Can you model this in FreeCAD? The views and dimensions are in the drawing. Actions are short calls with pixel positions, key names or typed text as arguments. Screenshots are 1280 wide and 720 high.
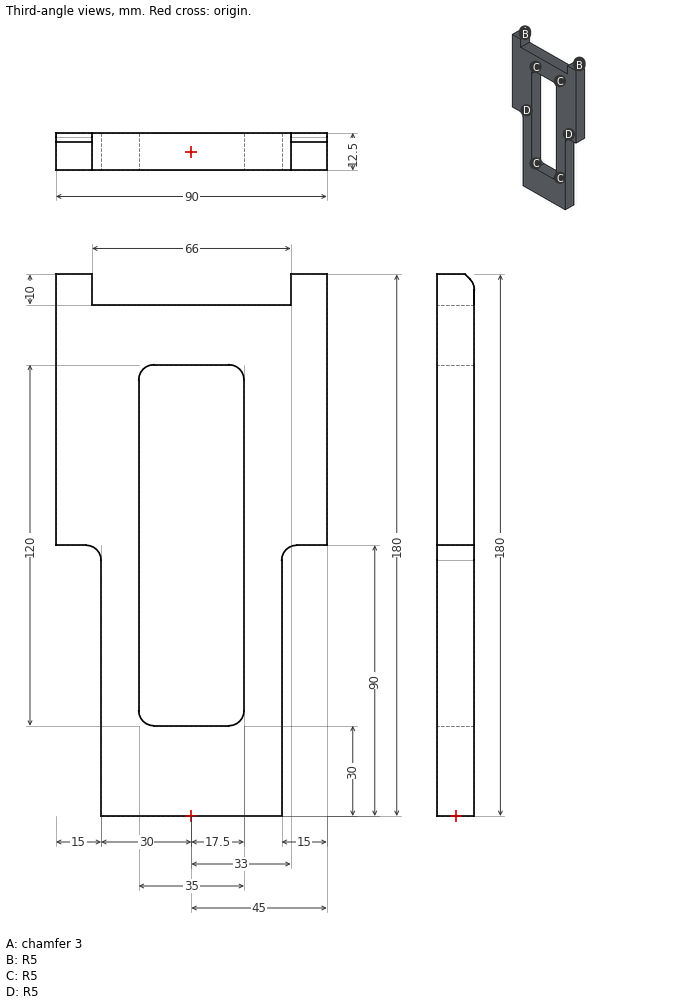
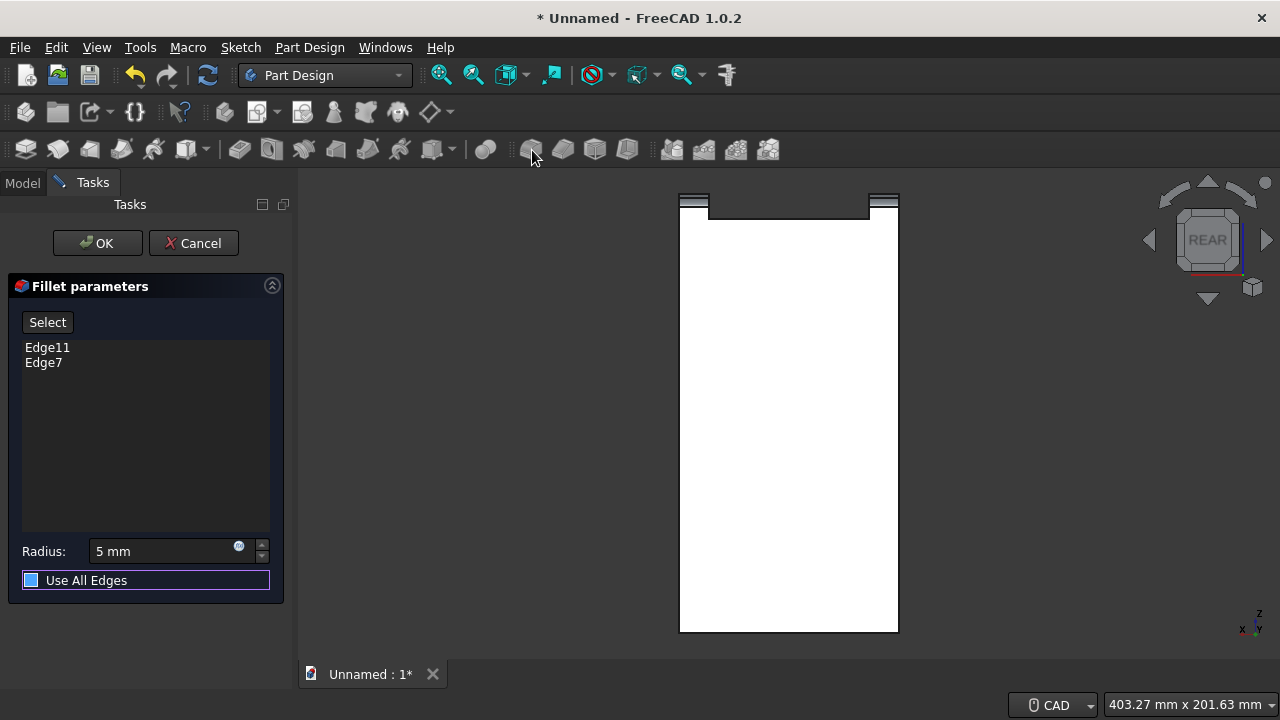
click(98, 243)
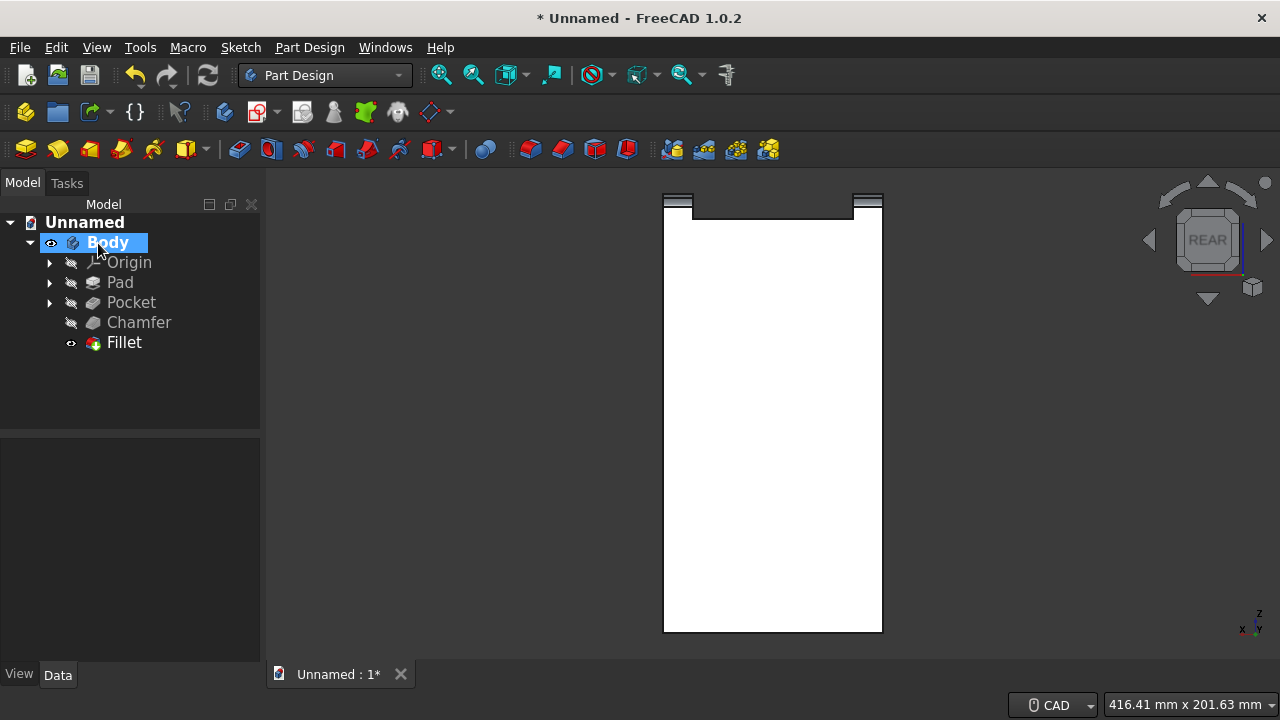
click(773, 358)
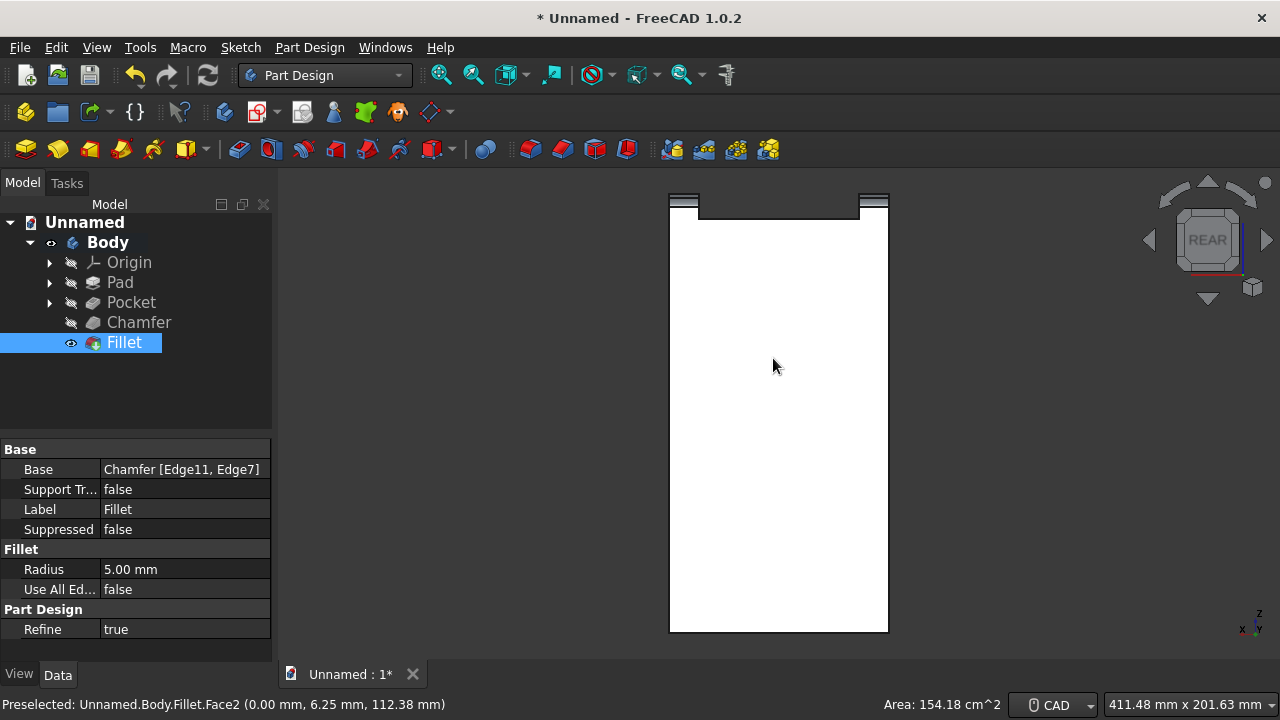
click(258, 112)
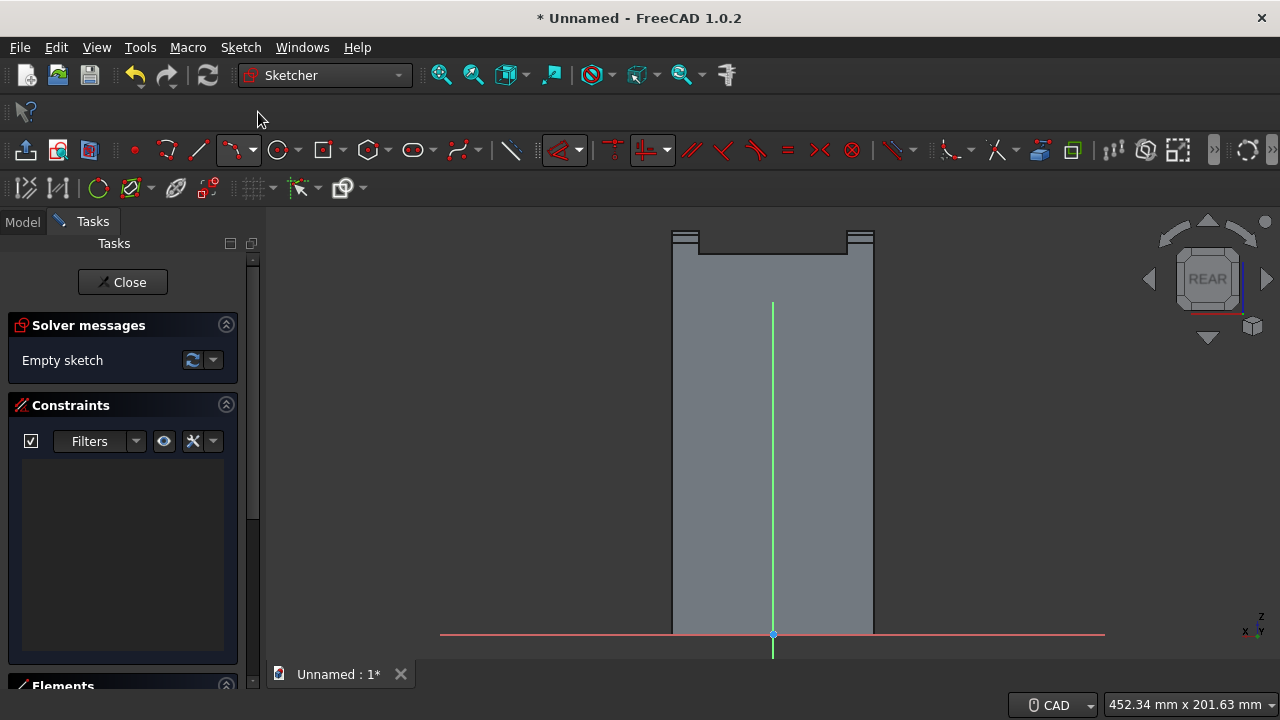
scroll(395, 235, down, 1)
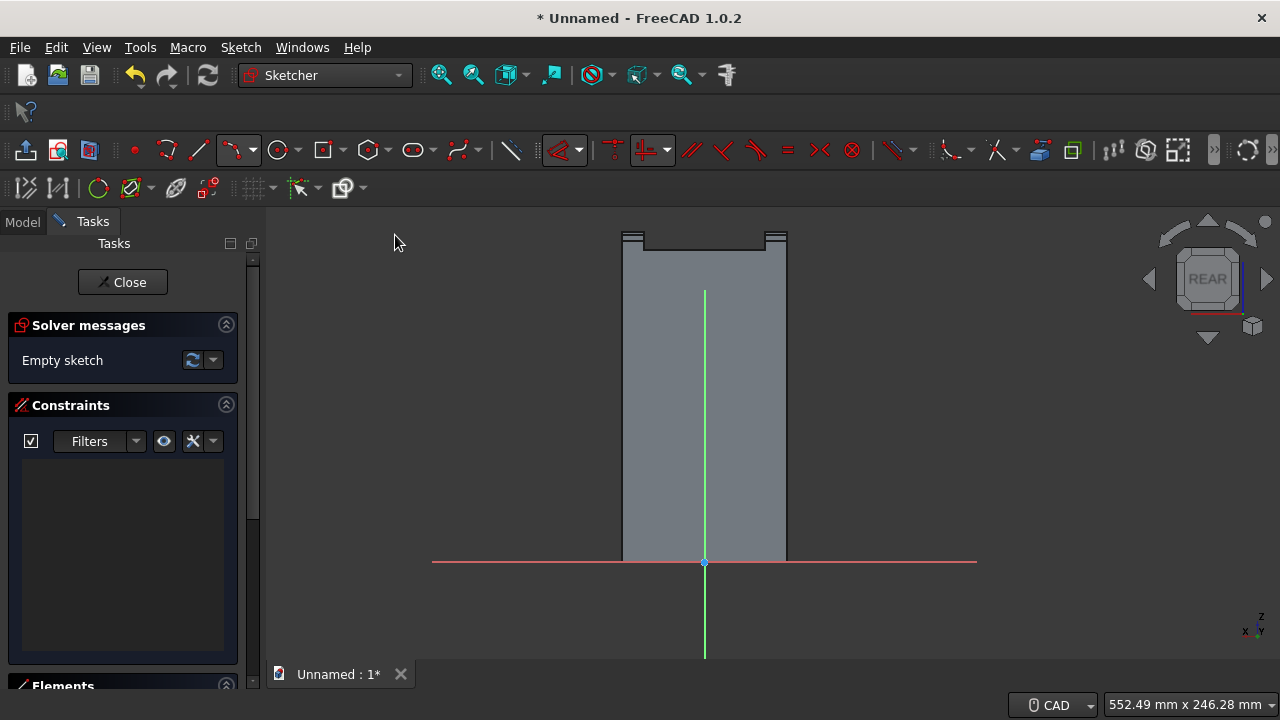
scroll(705, 537, up, 3)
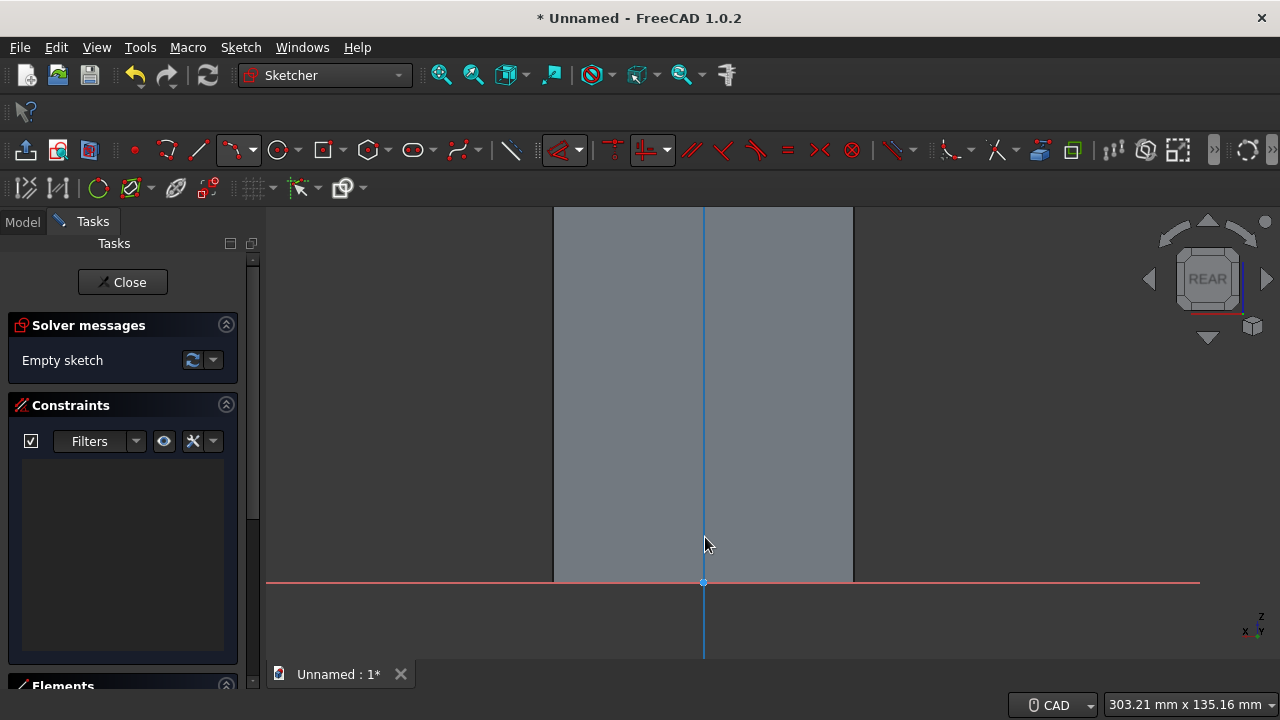
click(346, 150)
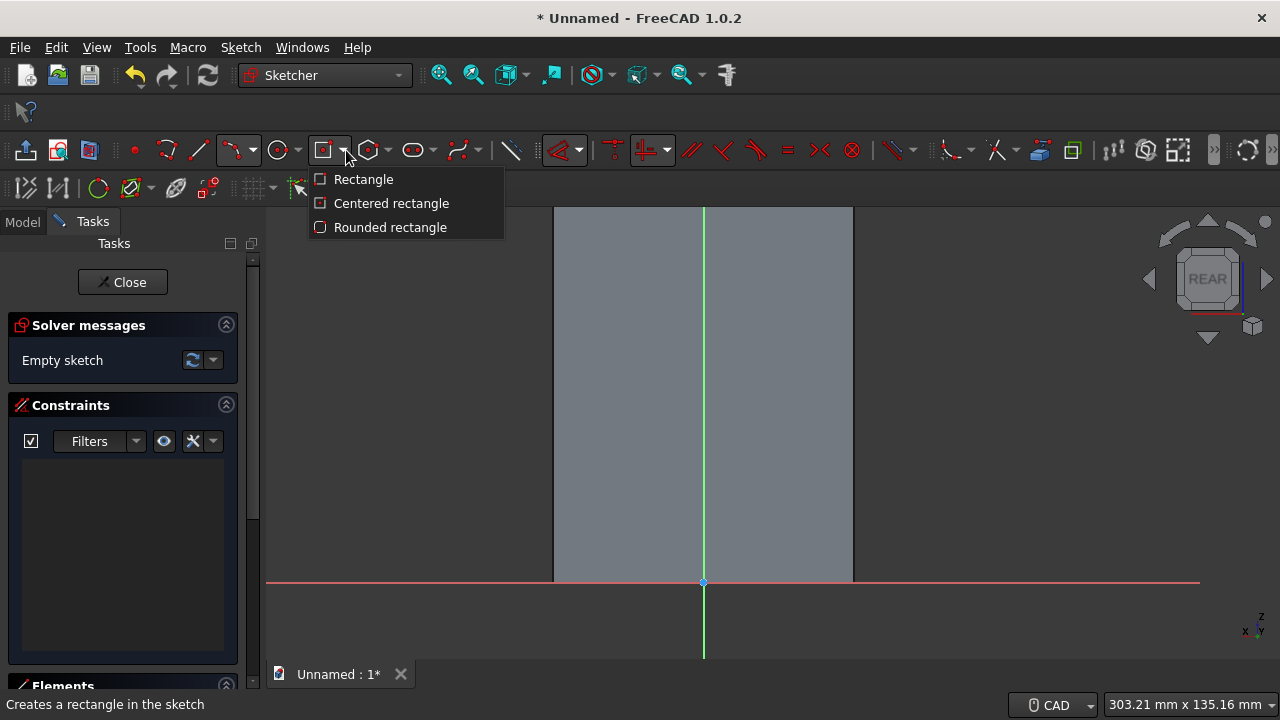
click(406, 179)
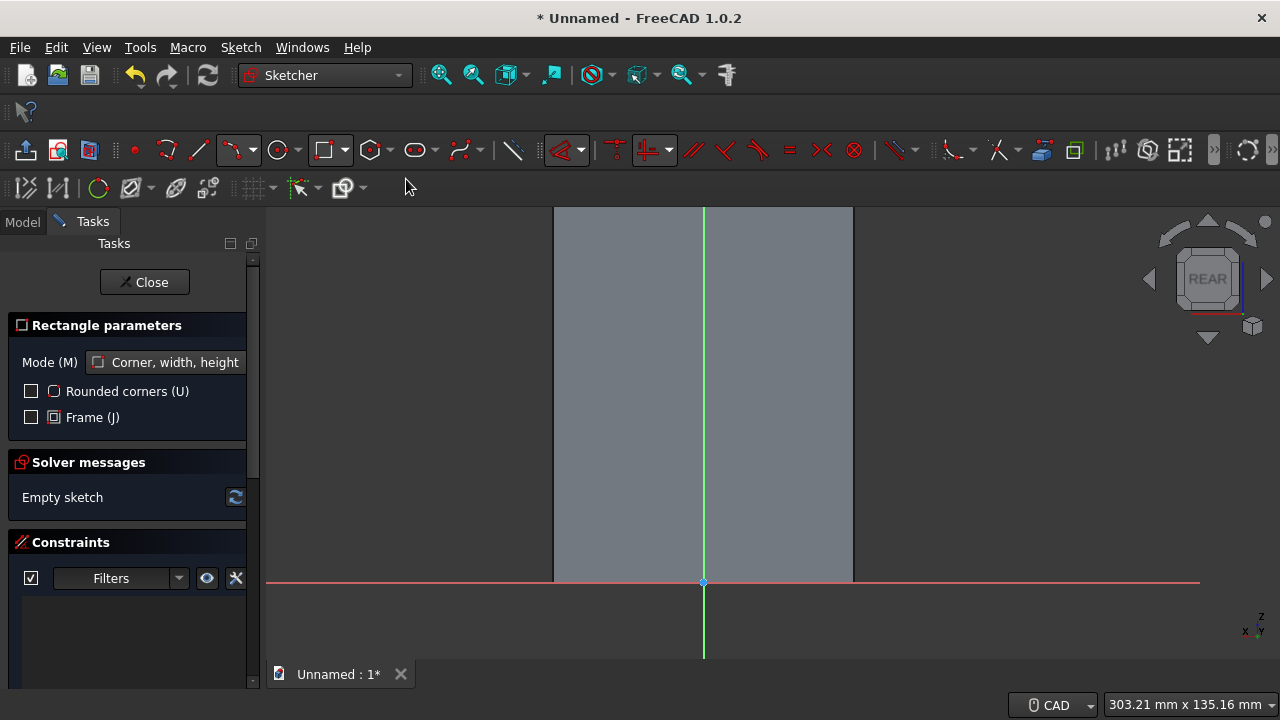
click(553, 282)
click(603, 582)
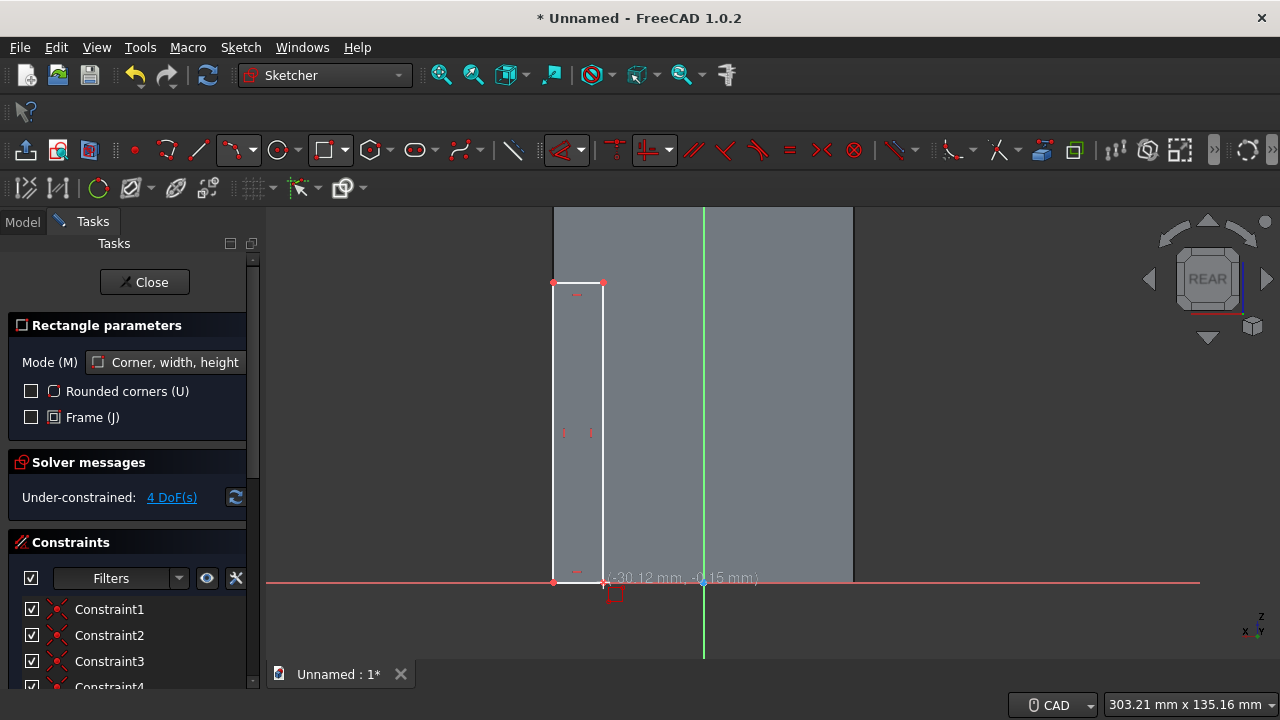
click(804, 282)
click(854, 582)
key(Escape)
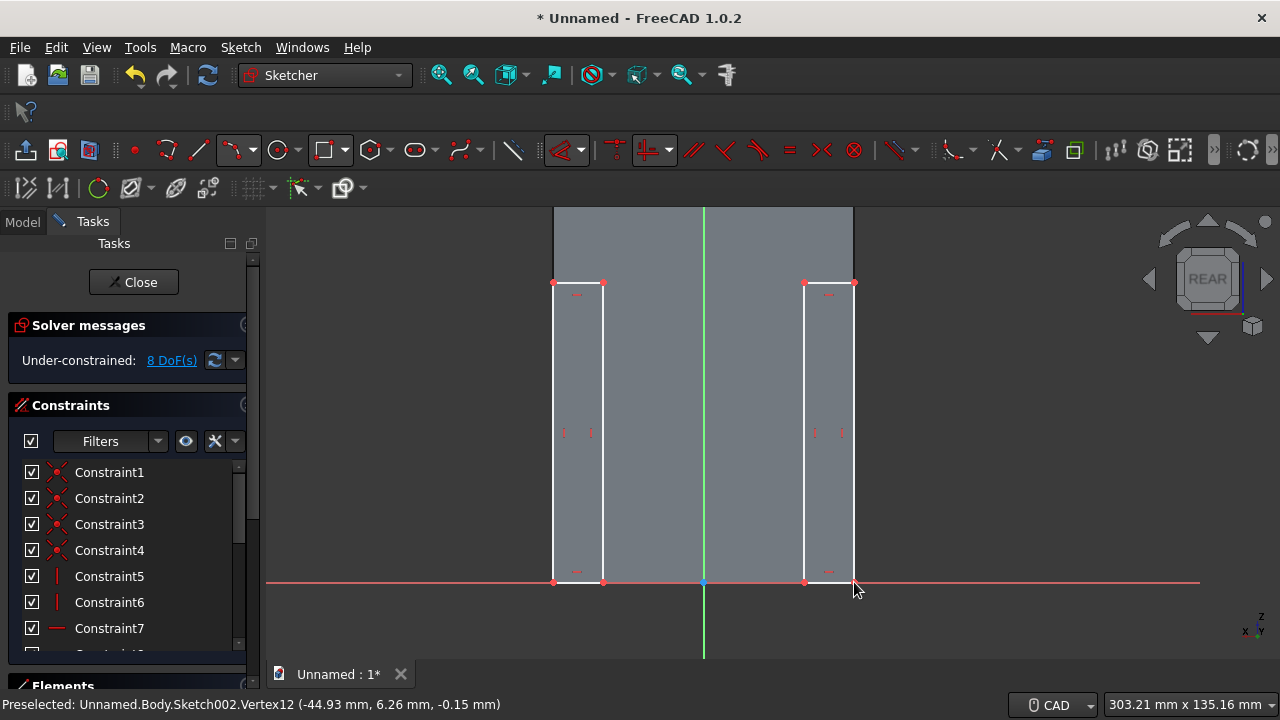
click(553, 583)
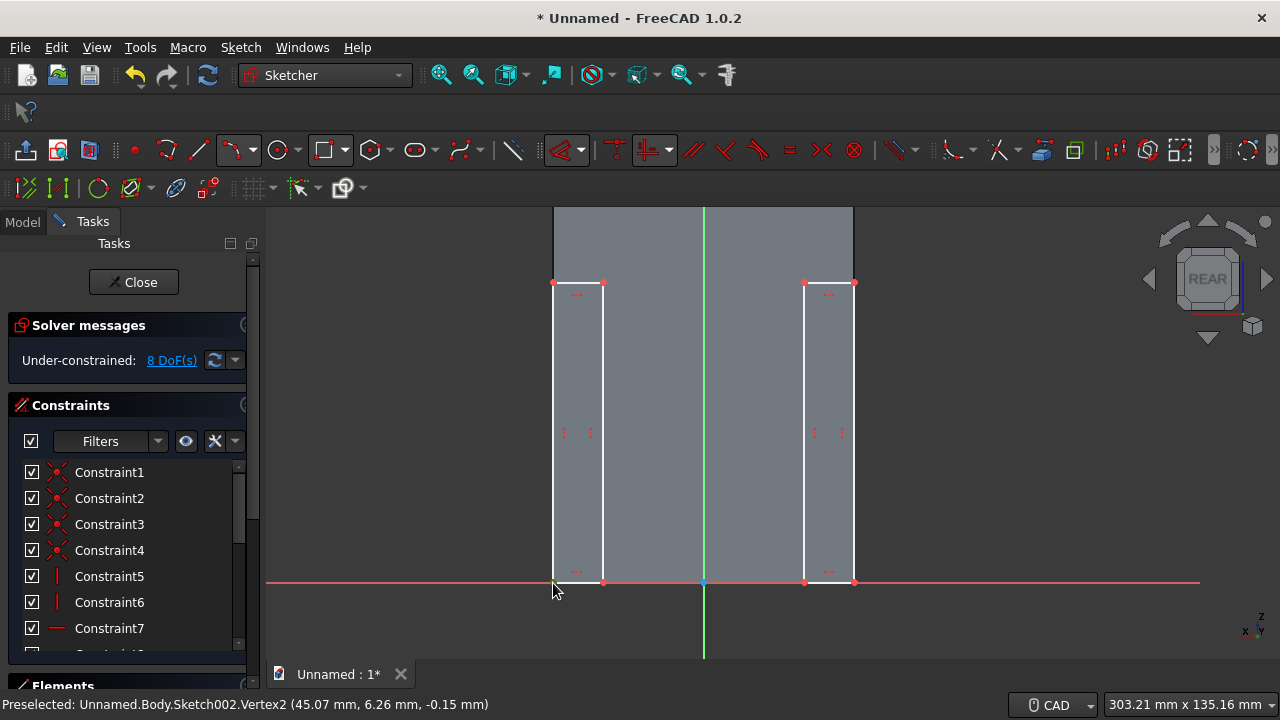
click(353, 582)